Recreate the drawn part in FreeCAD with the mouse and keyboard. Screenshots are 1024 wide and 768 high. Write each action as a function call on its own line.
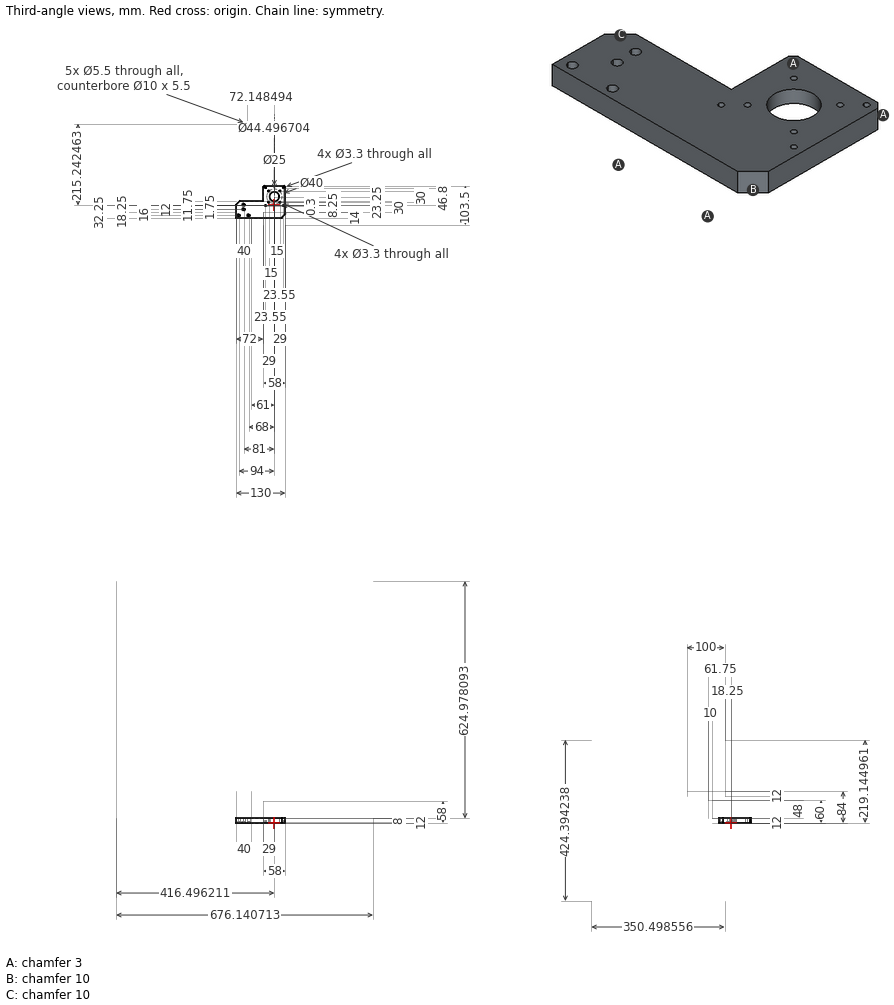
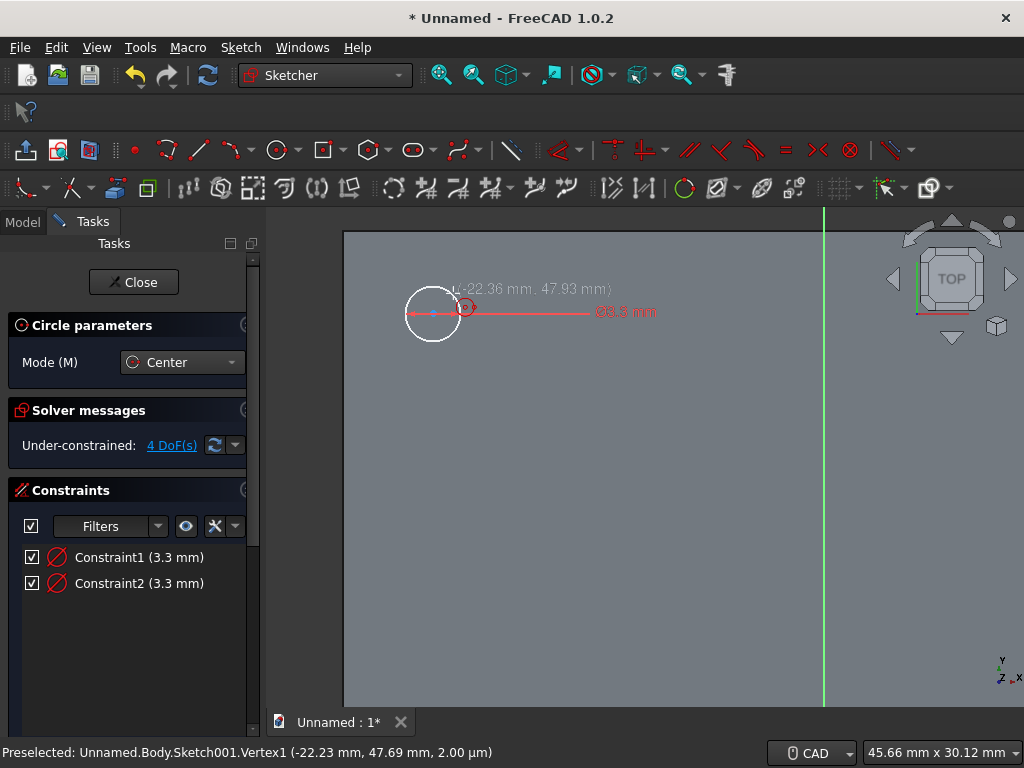
scroll(432, 313, down, 5)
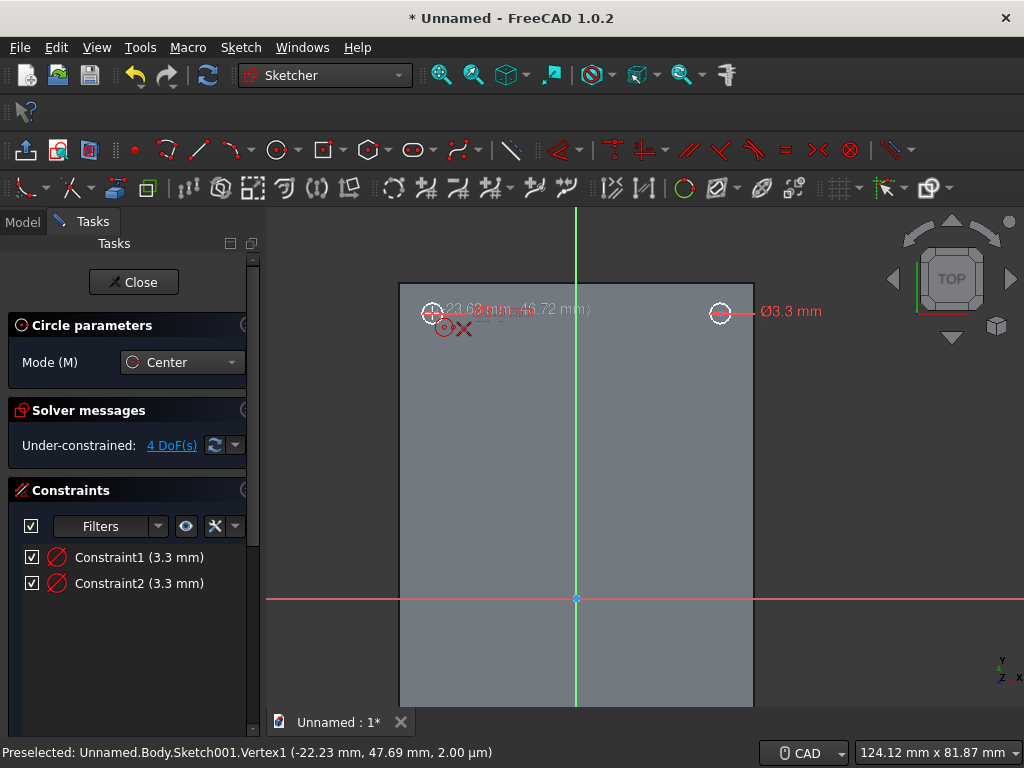
scroll(433, 601, up, 11)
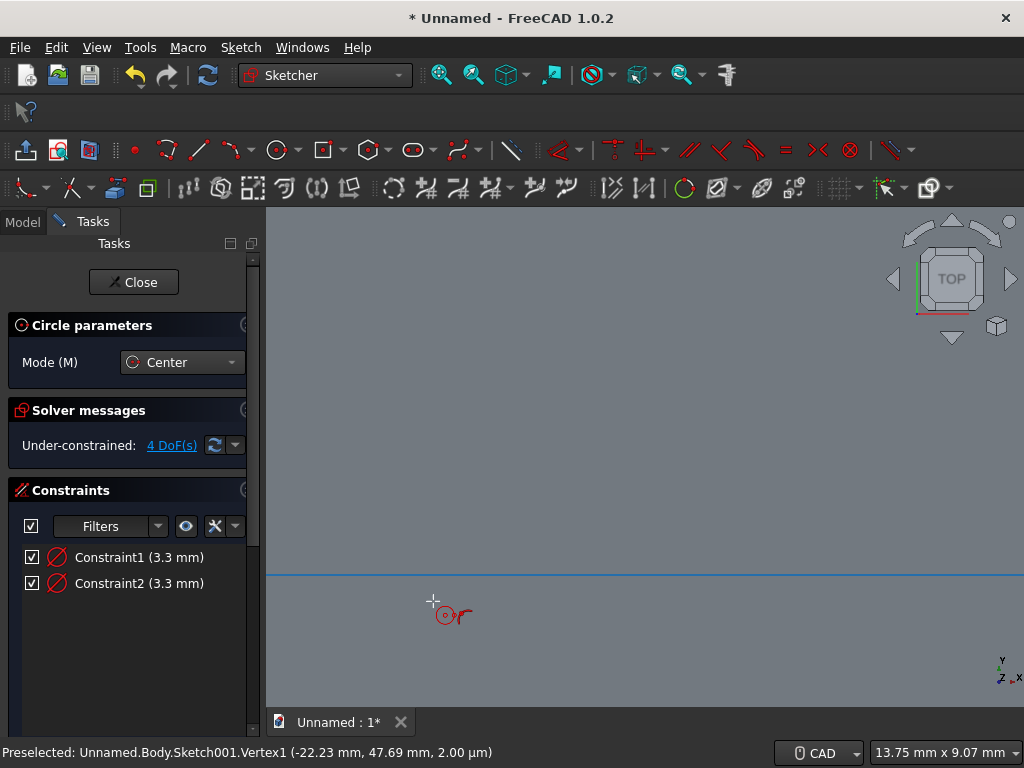
click(428, 592)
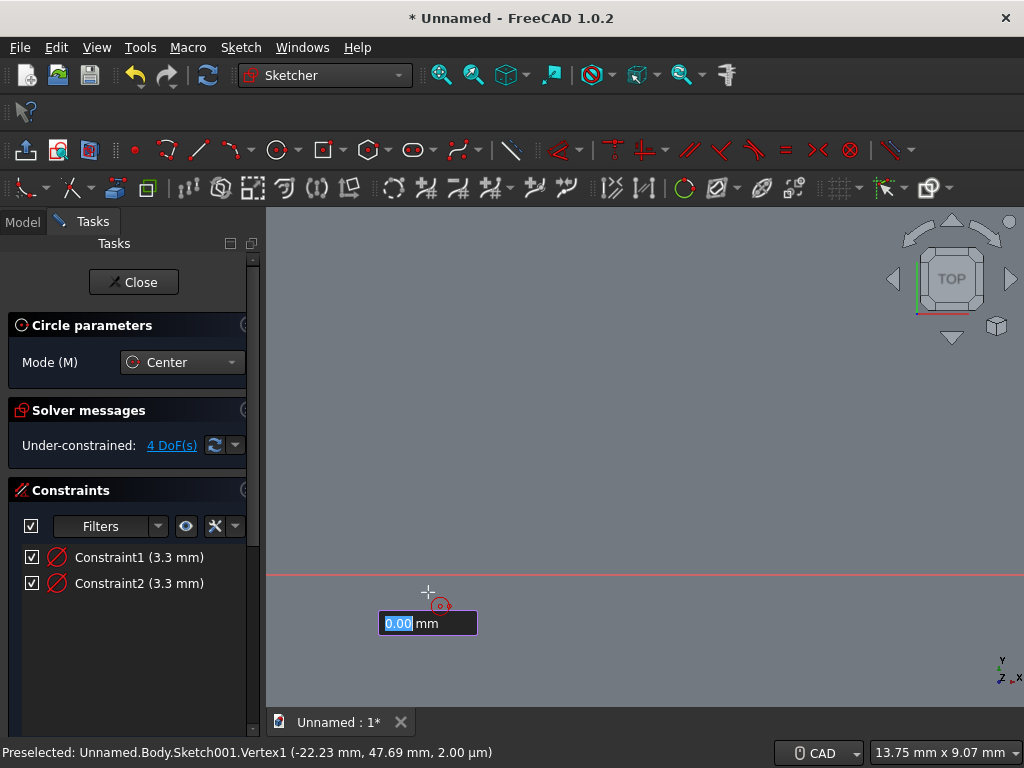
scroll(433, 602, down, 11)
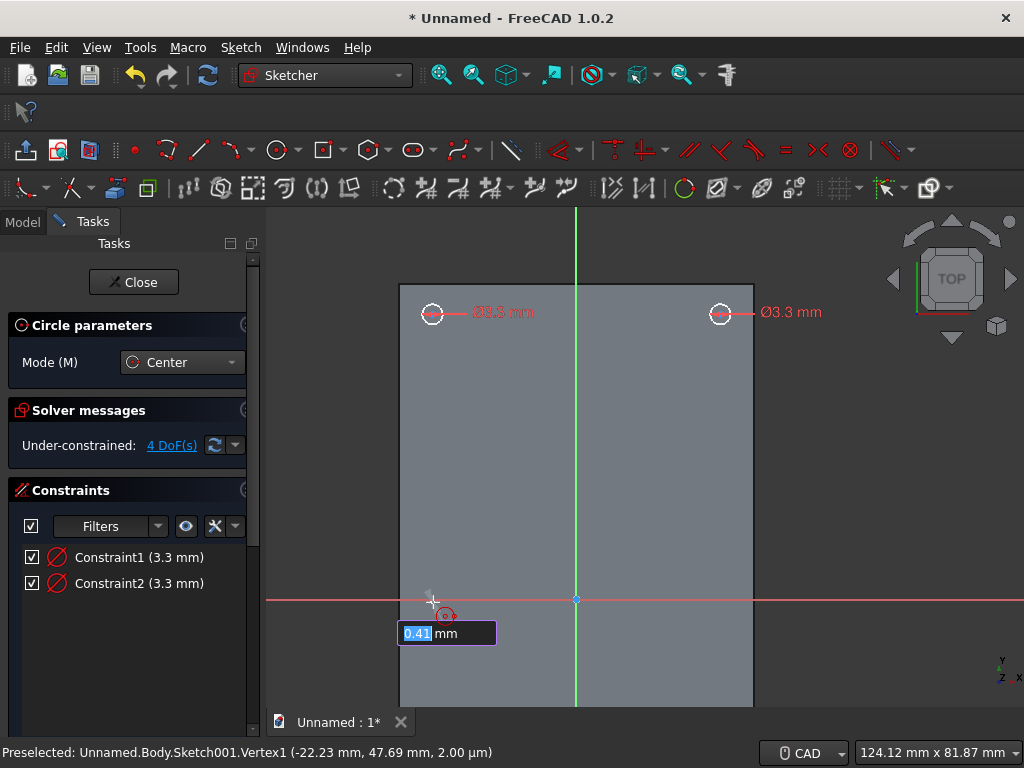
scroll(440, 594, up, 6)
move(439, 594)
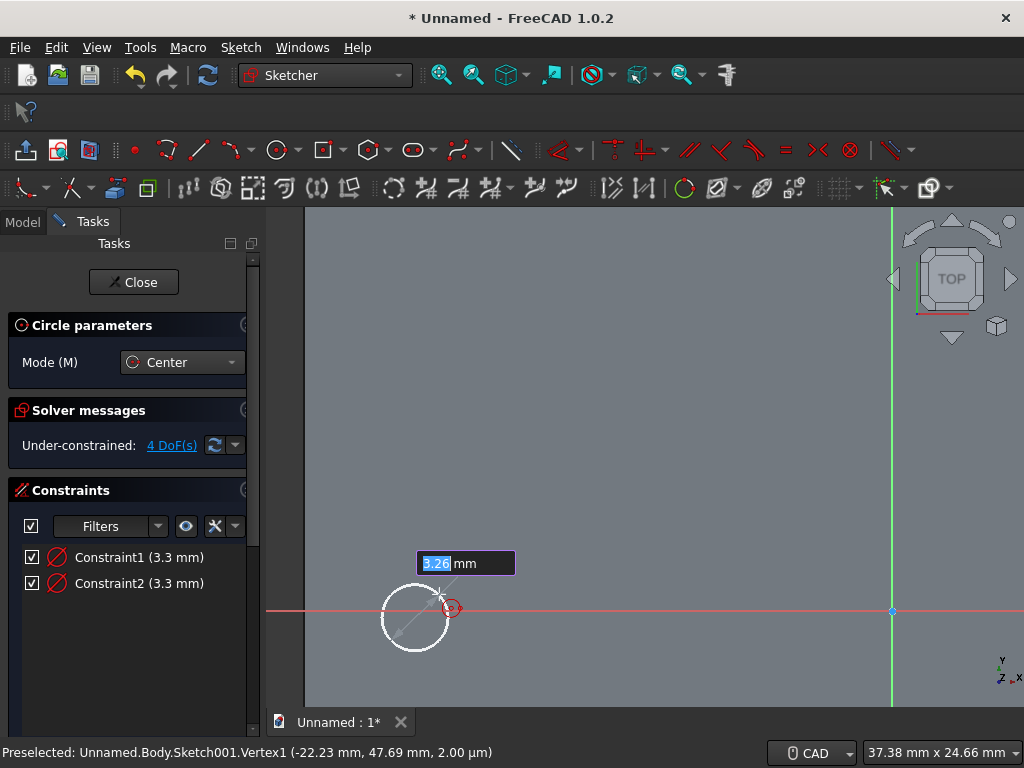
text(3.3)
key(Return)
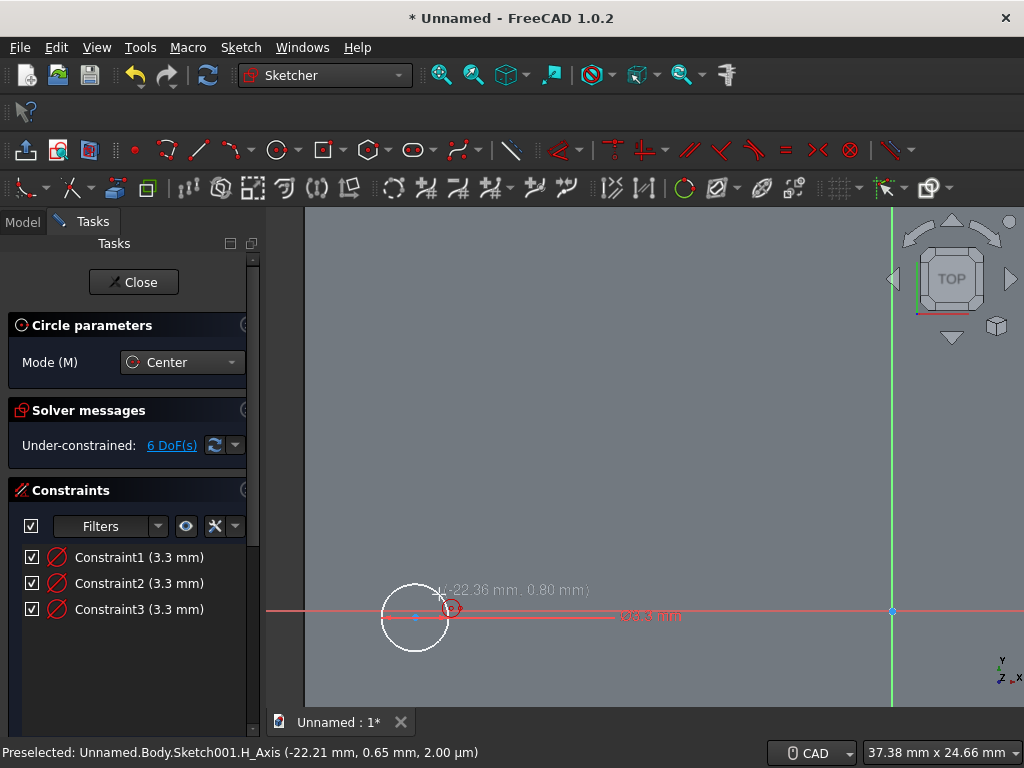
scroll(440, 594, down, 6)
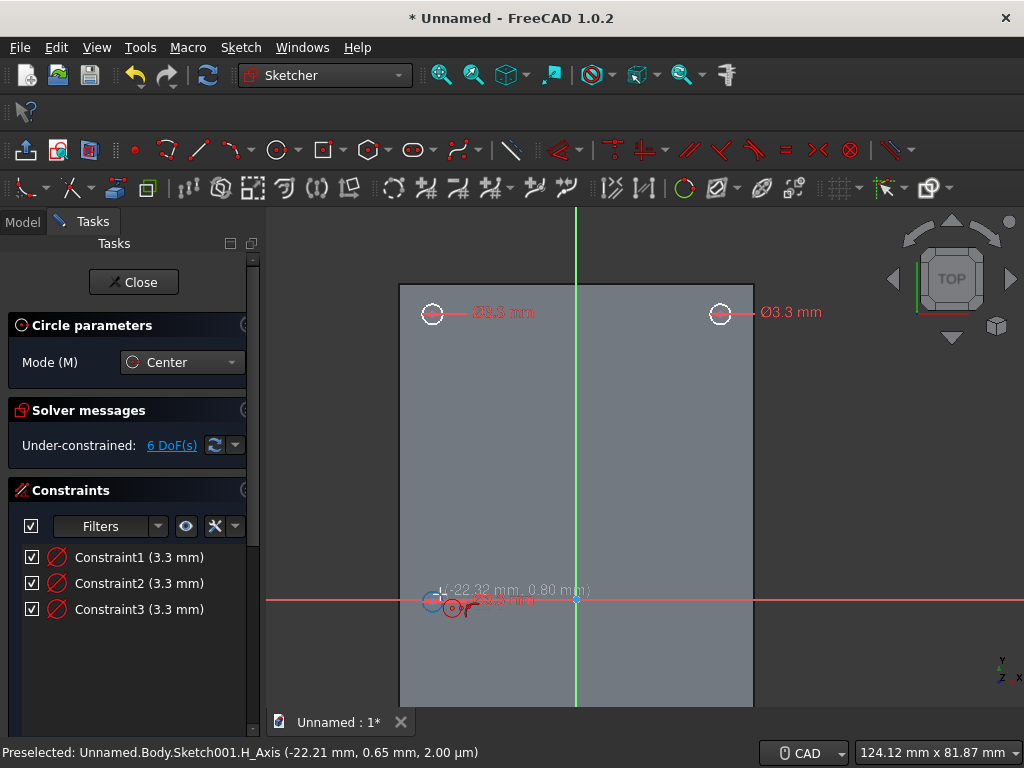
scroll(720, 602, up, 11)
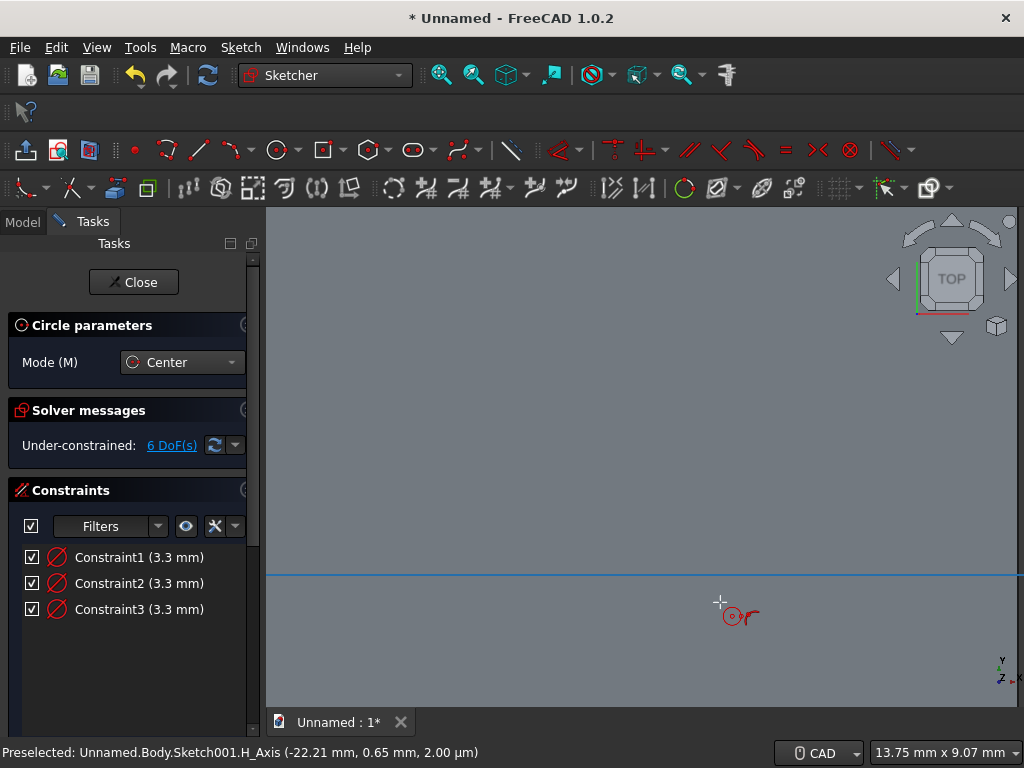
click(718, 592)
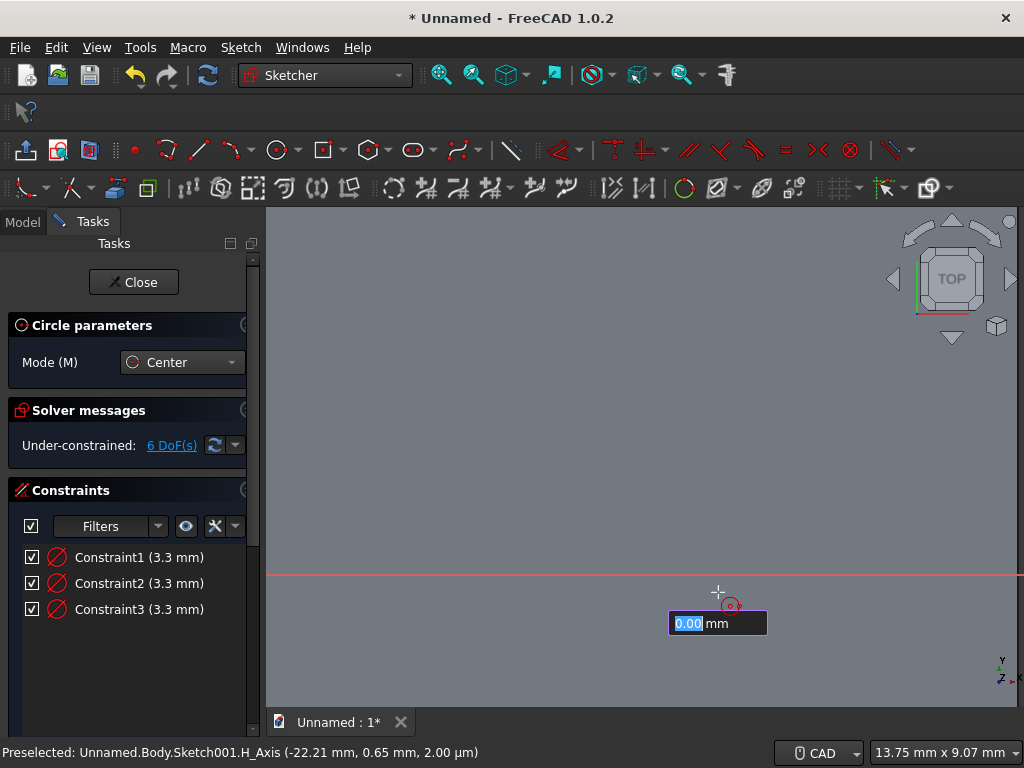
scroll(721, 602, down, 11)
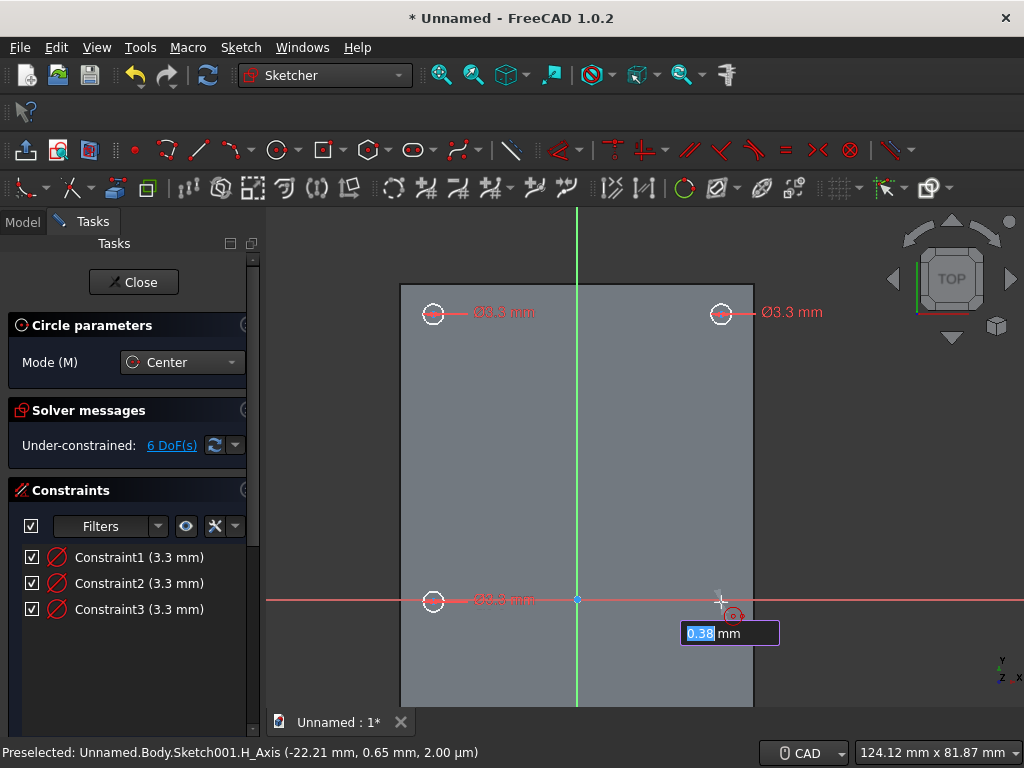
scroll(728, 594, up, 6)
move(727, 594)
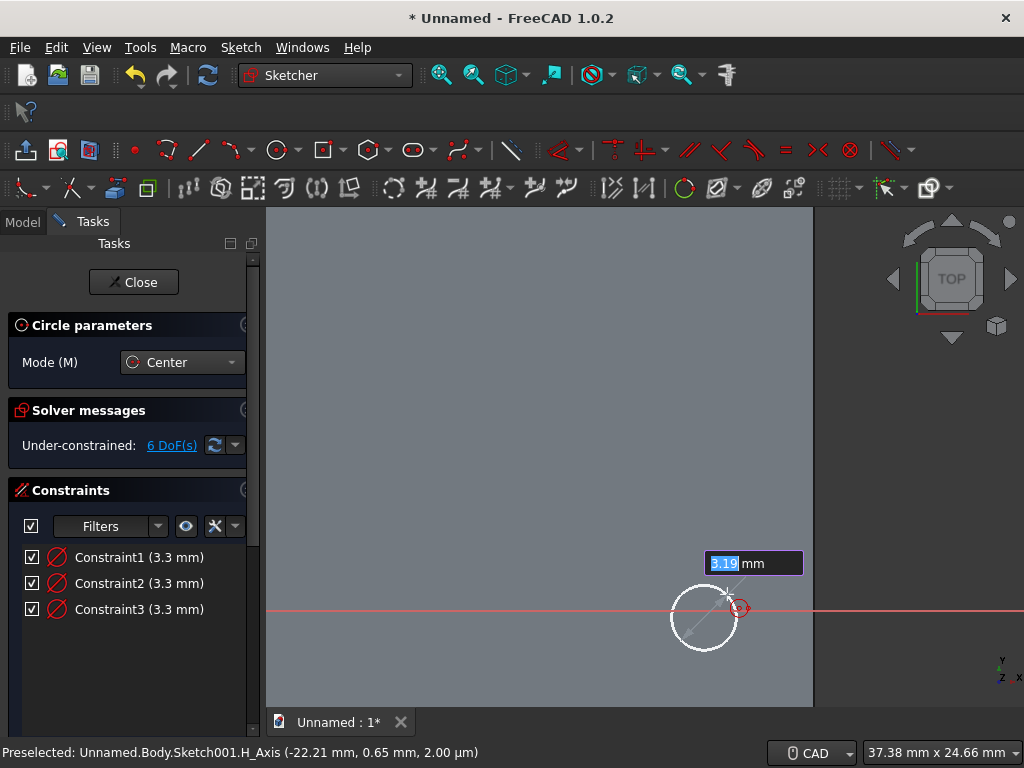
text(3.3)
key(Return)
key(Escape)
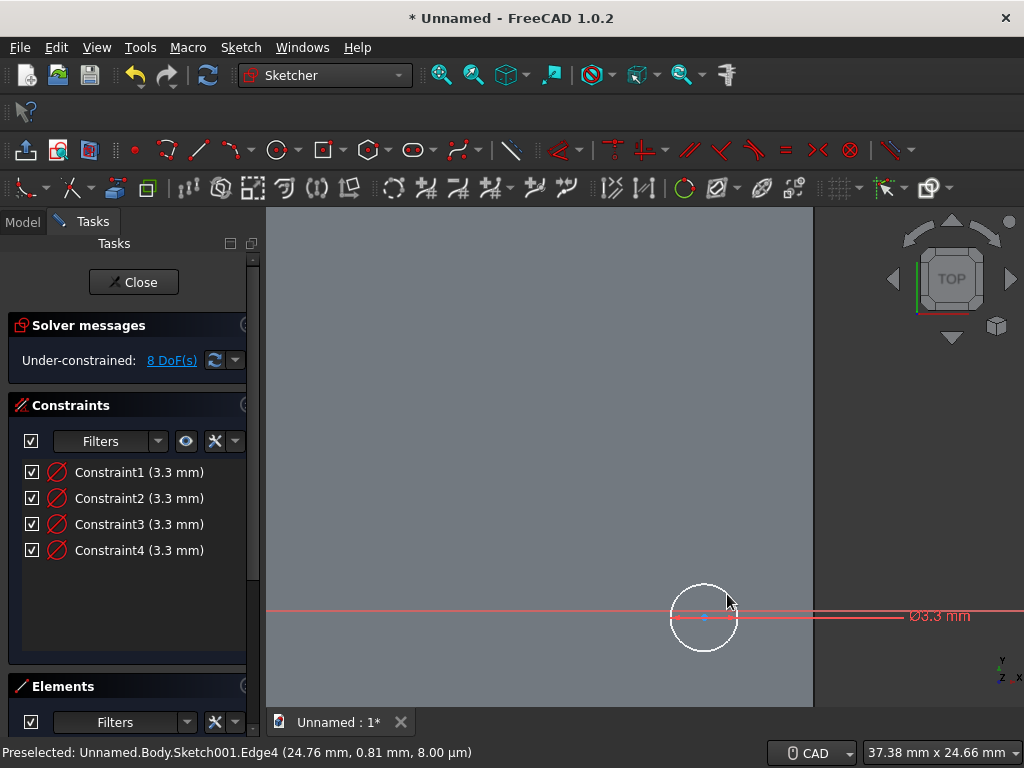
scroll(727, 594, down, 6)